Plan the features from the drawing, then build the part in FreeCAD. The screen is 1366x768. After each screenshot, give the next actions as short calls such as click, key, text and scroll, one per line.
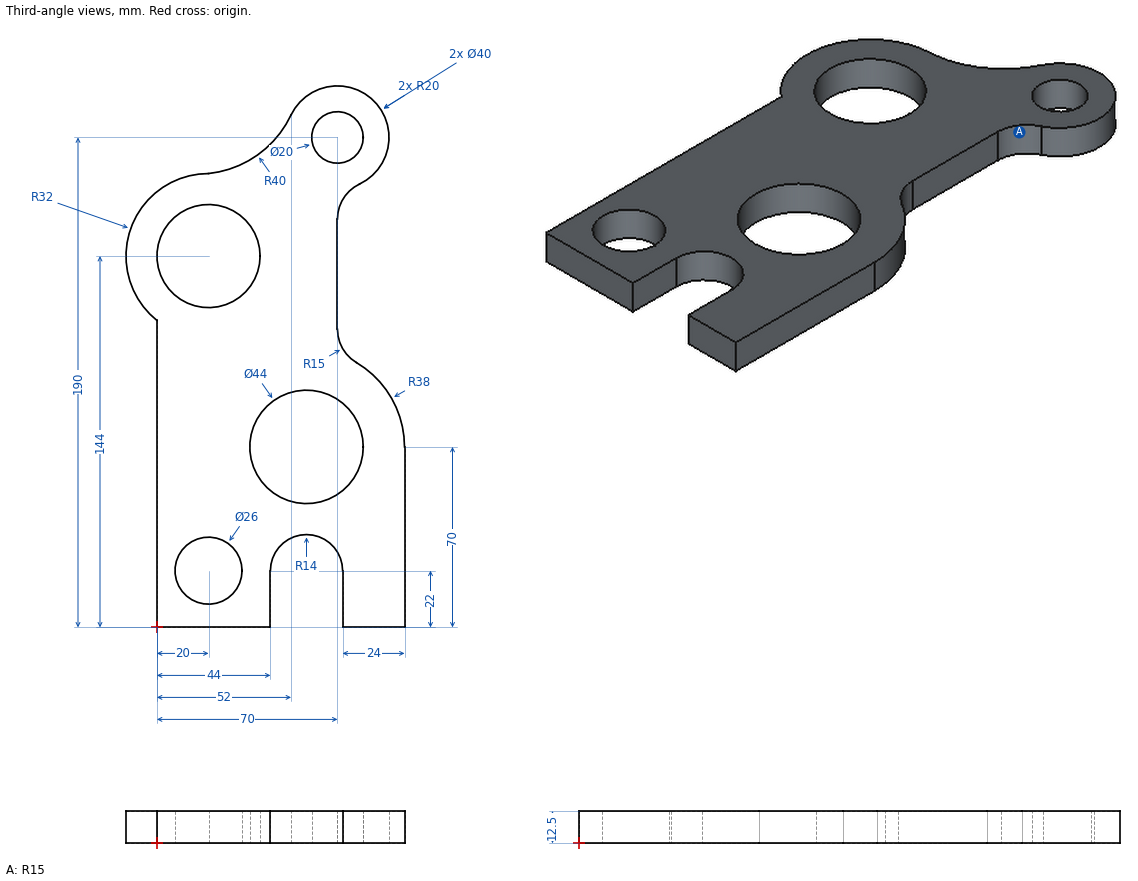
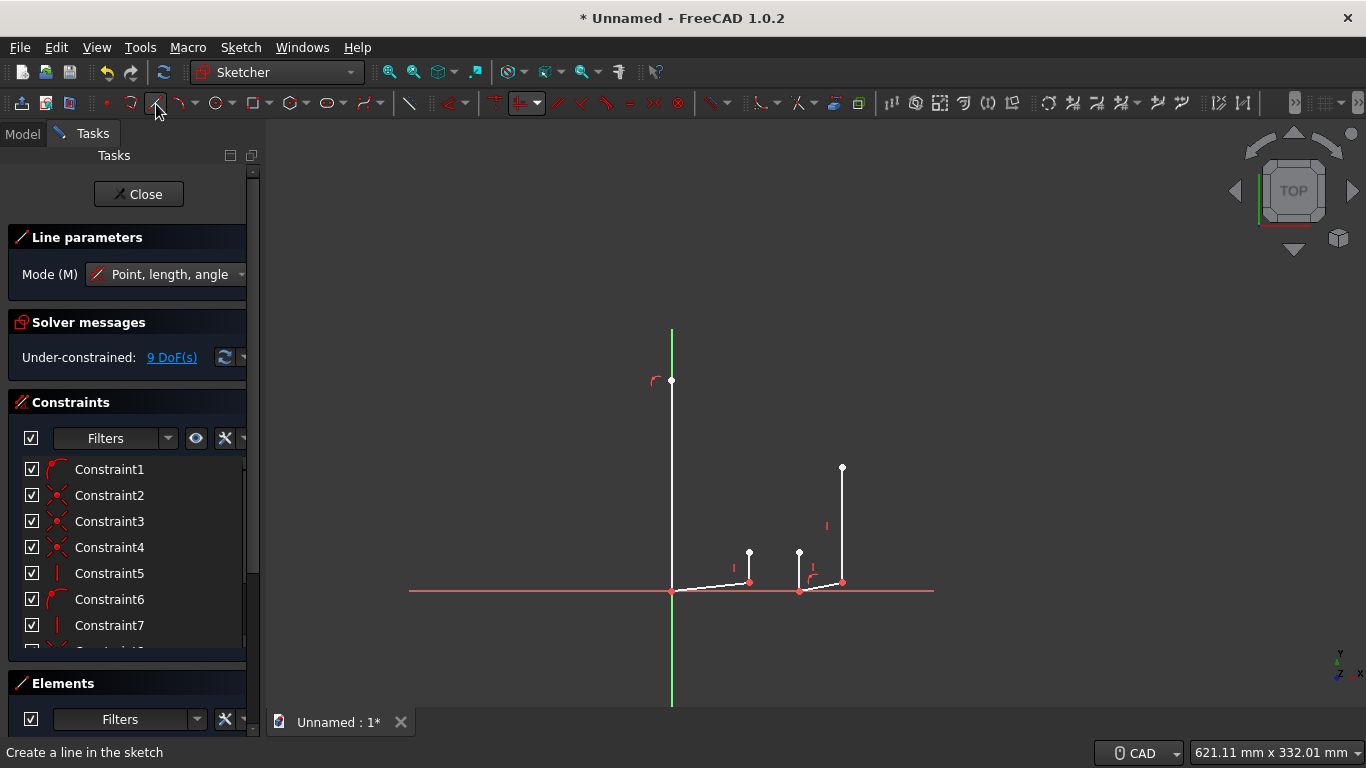
click(796, 386)
click(796, 290)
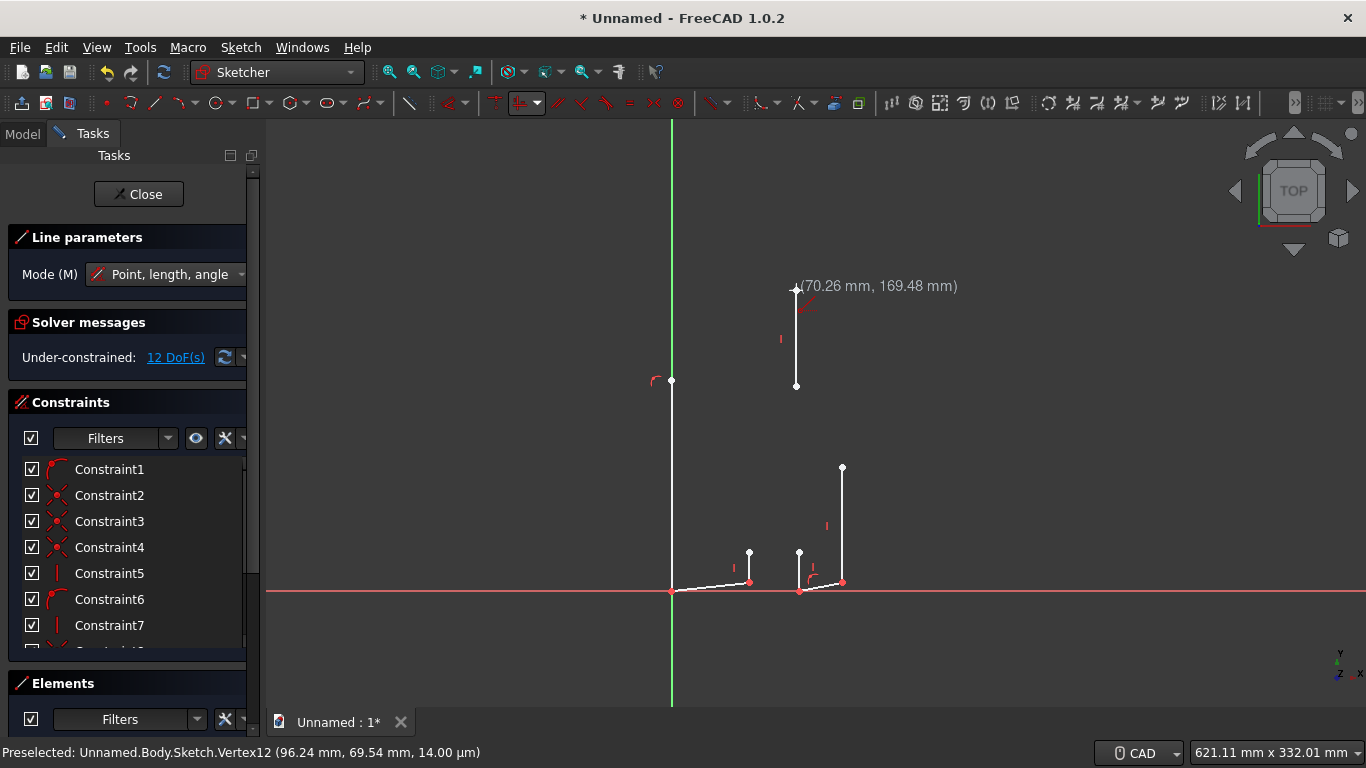
click(180, 104)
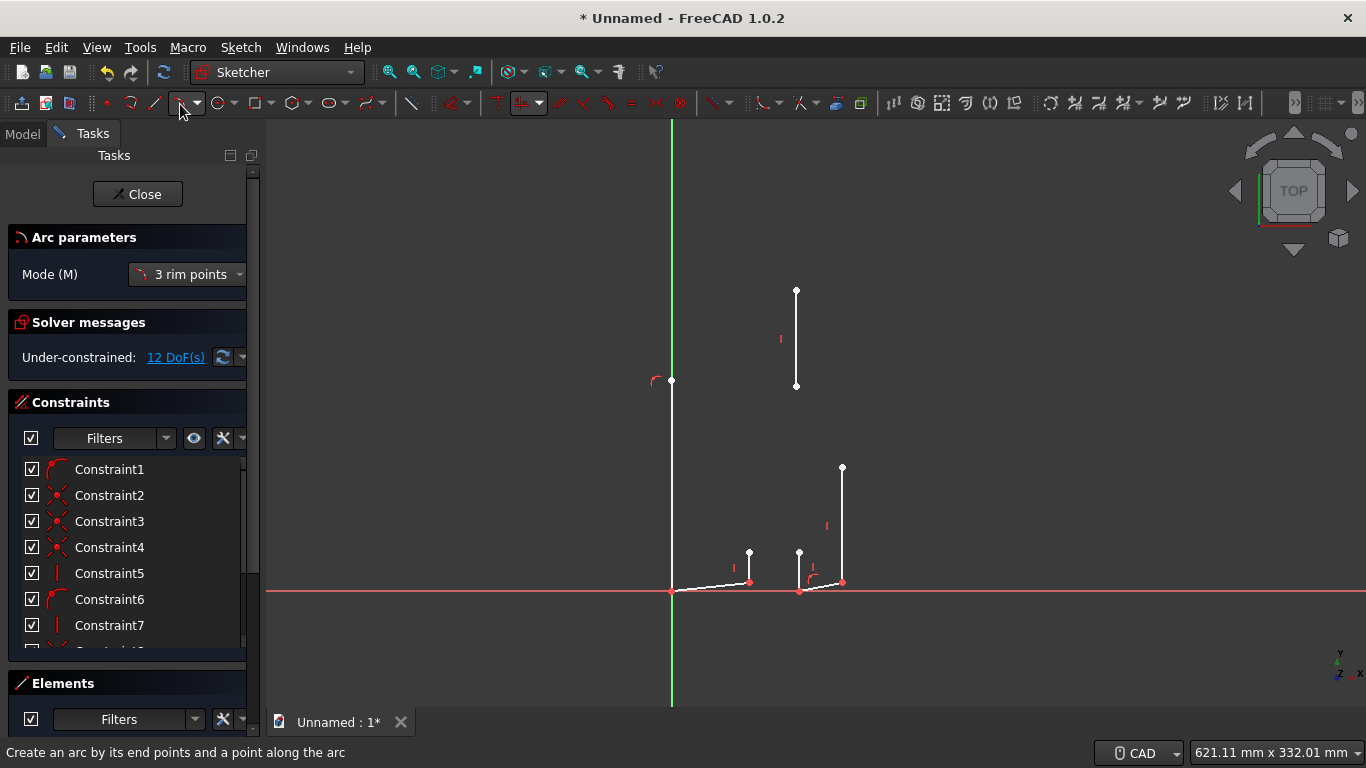
click(749, 553)
click(799, 553)
click(774, 527)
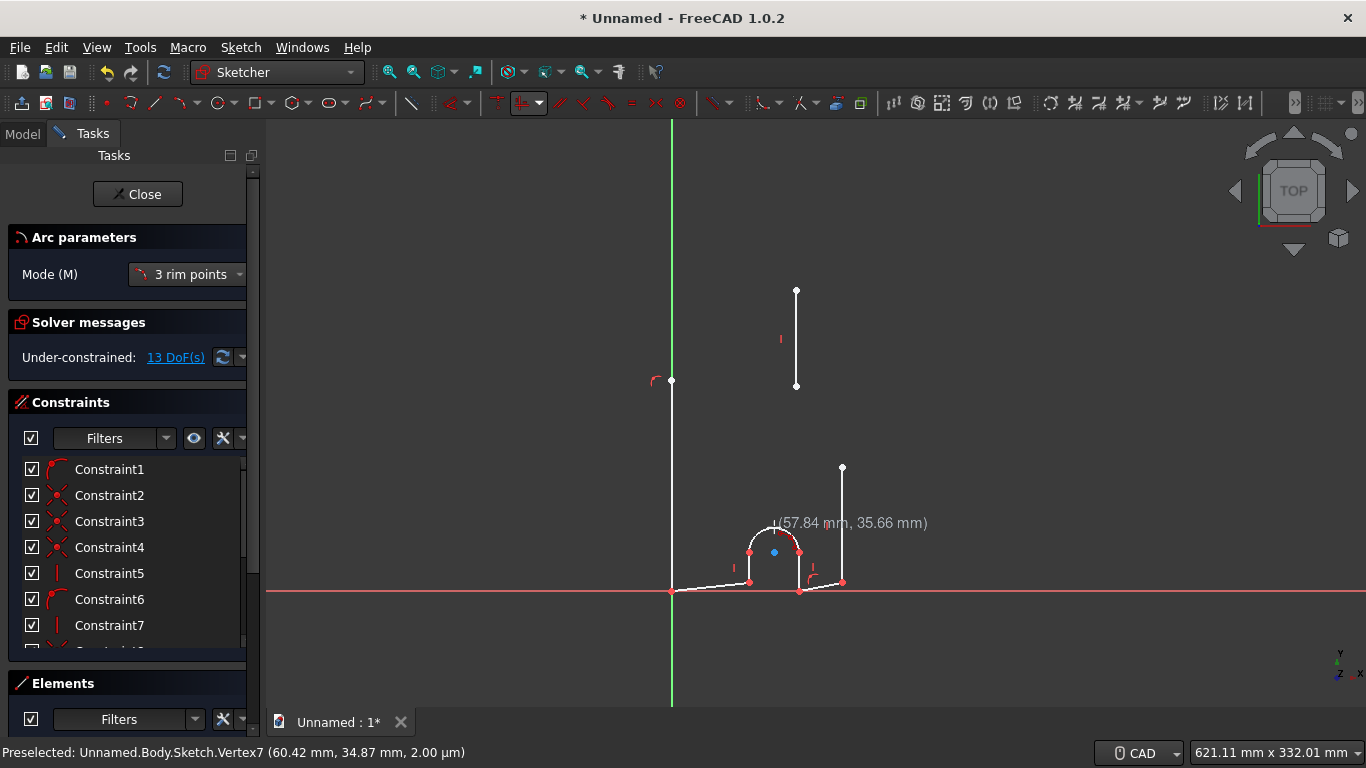
click(842, 468)
click(809, 409)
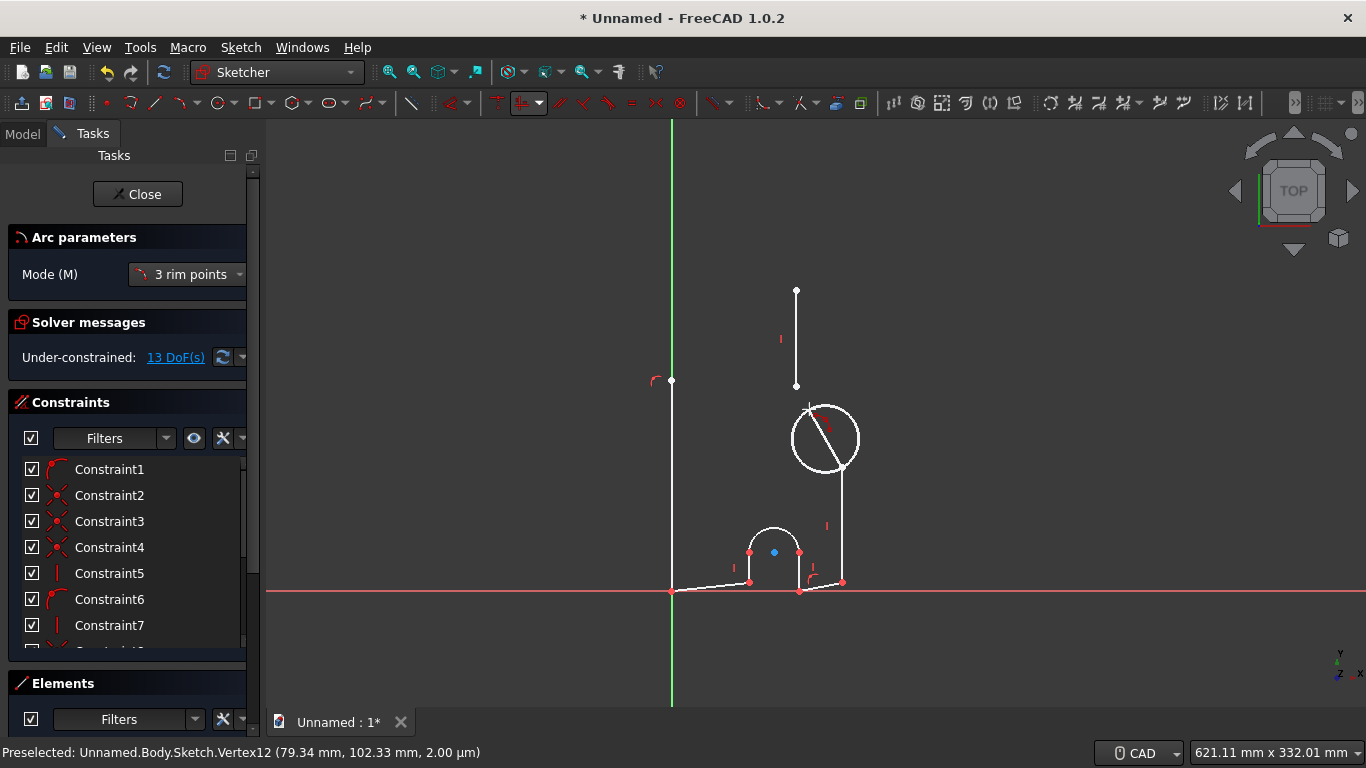
scroll(833, 434, up, 3)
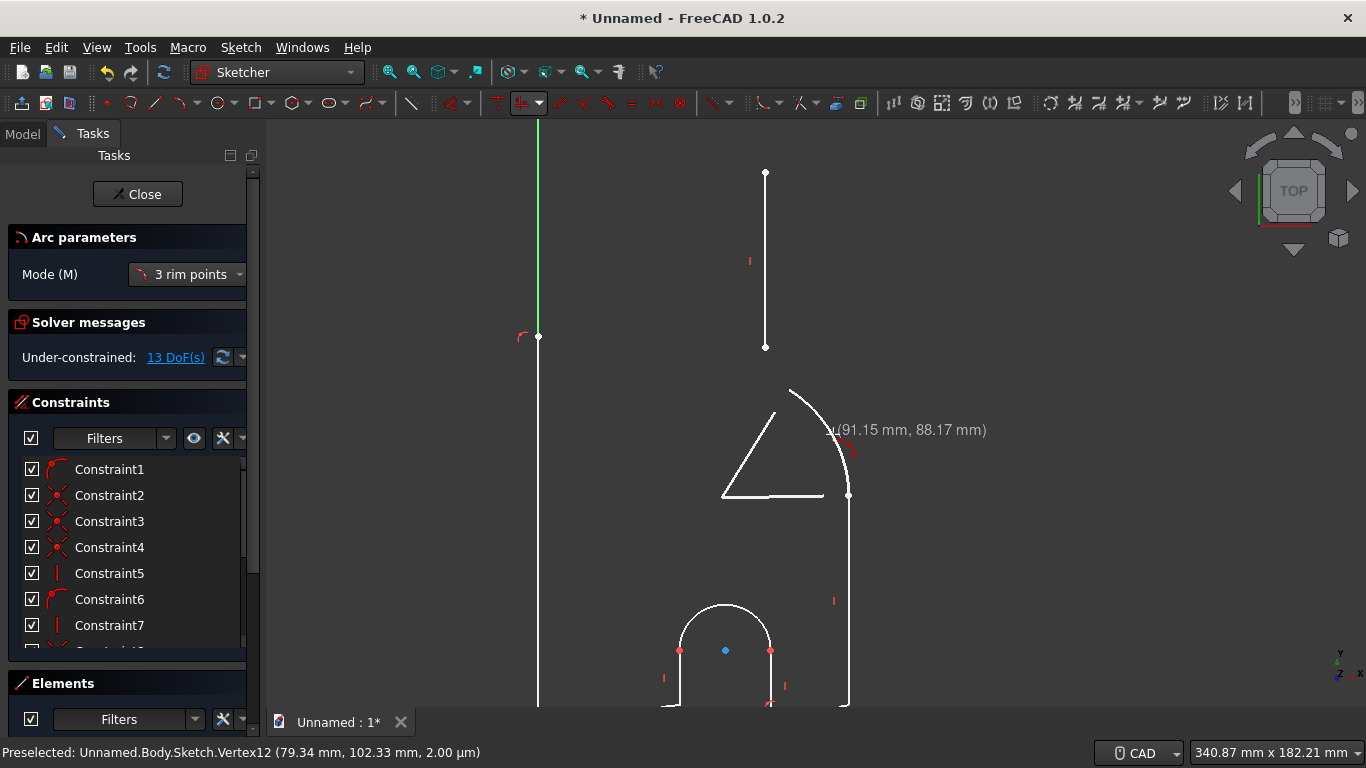
click(832, 433)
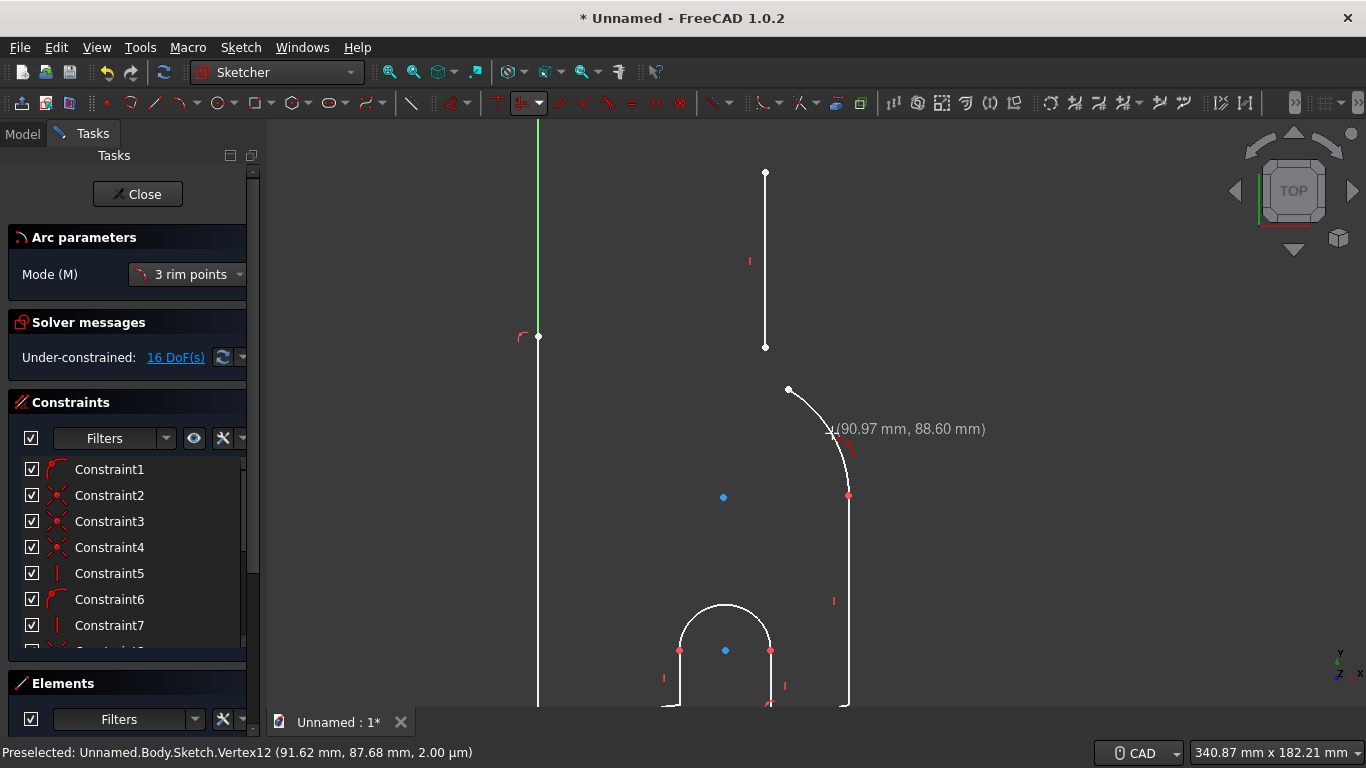
click(789, 390)
click(765, 348)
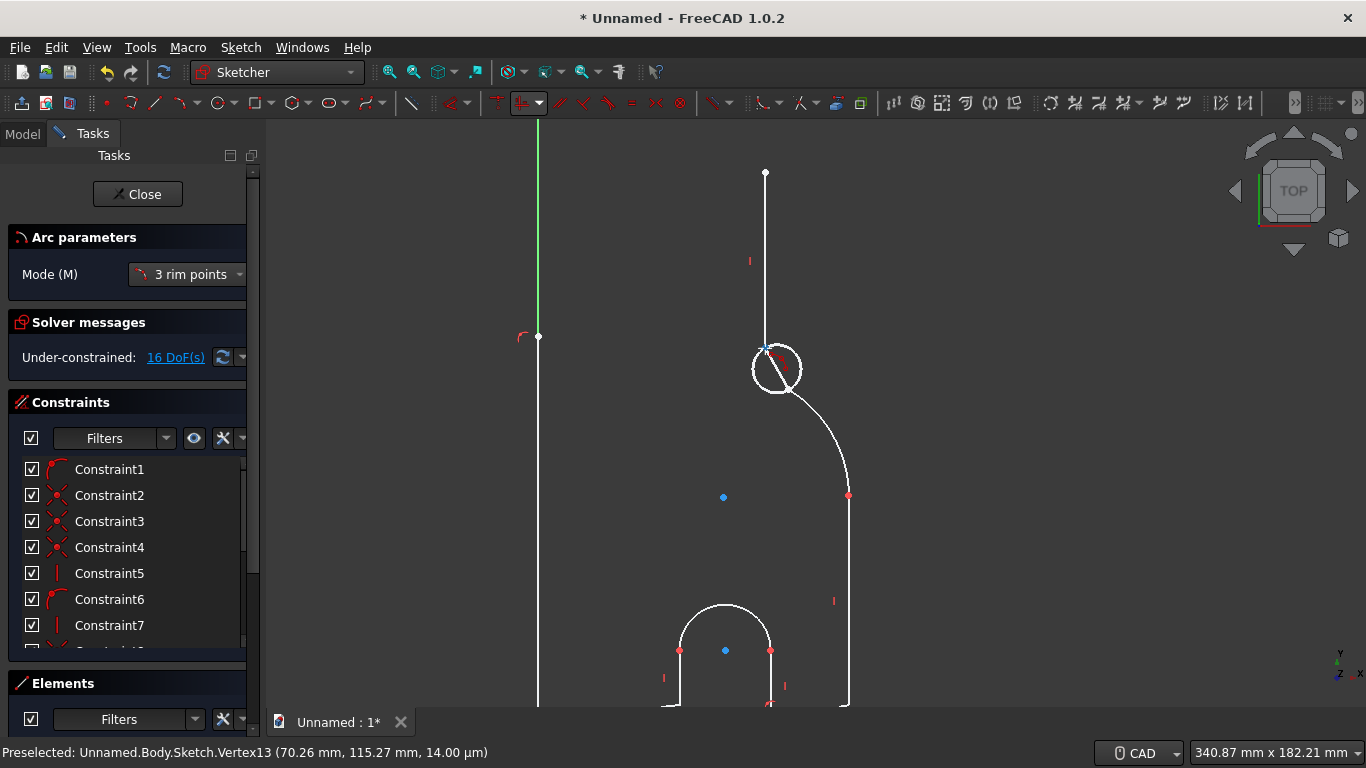
scroll(771, 371, up, 5)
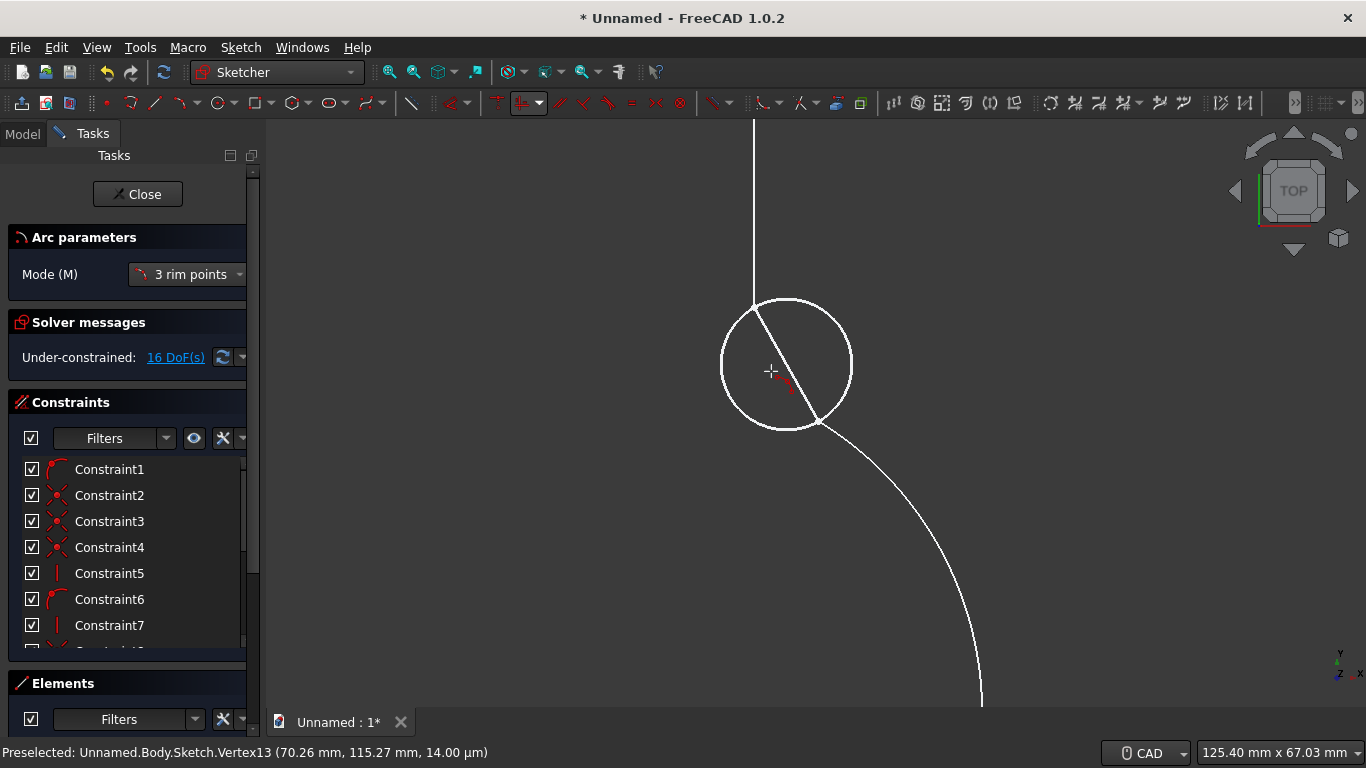
click(769, 370)